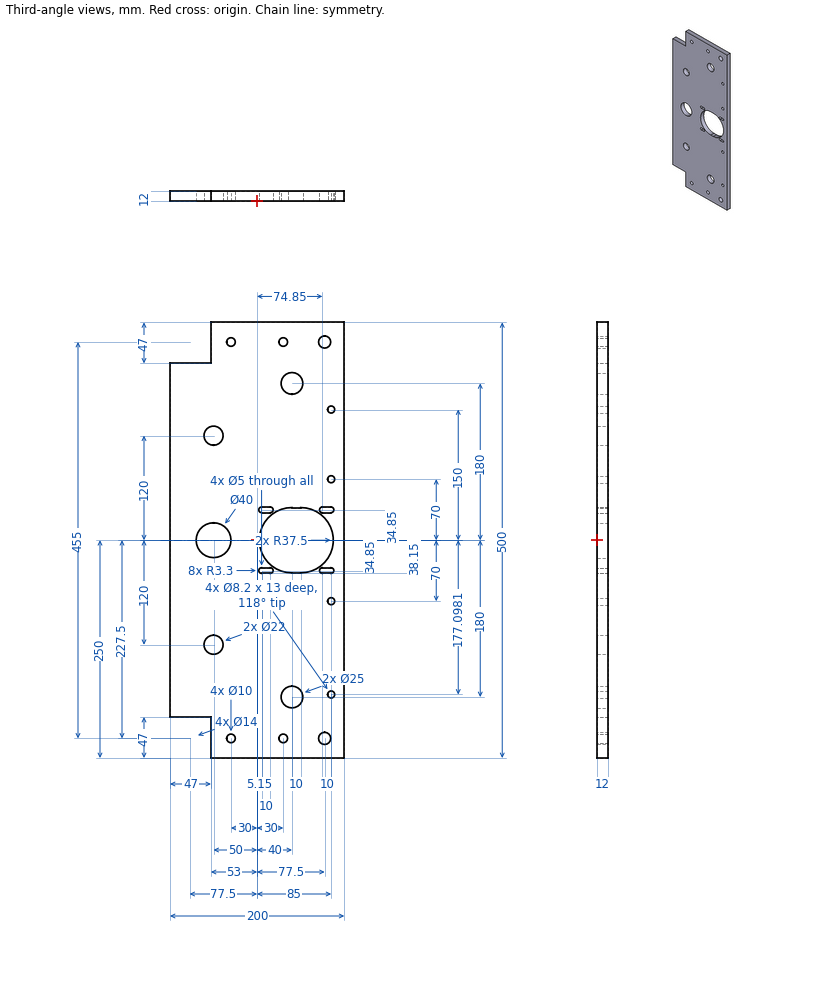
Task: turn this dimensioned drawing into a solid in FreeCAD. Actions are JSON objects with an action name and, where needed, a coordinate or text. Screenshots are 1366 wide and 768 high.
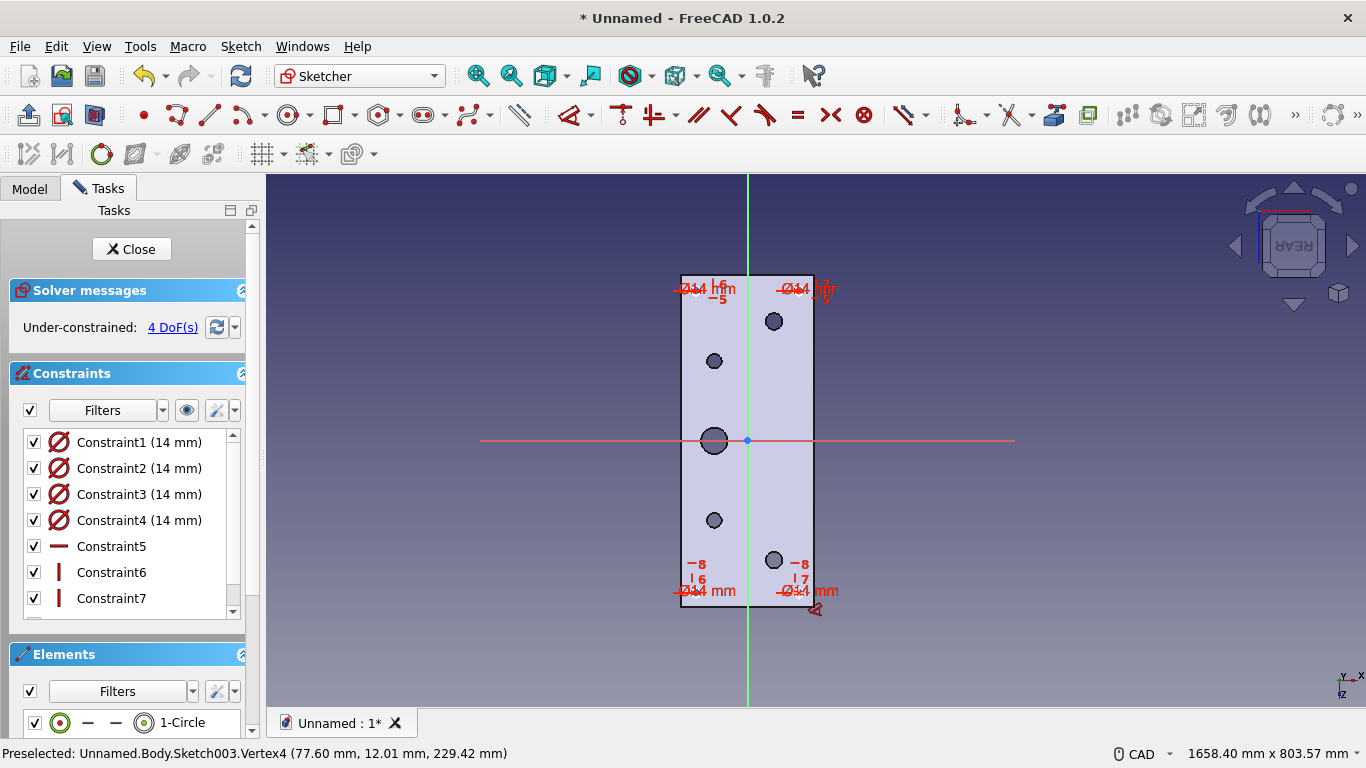
{"action": "left_click", "coordinate": [696, 291]}
{"action": "left_click", "coordinate": [722, 257]}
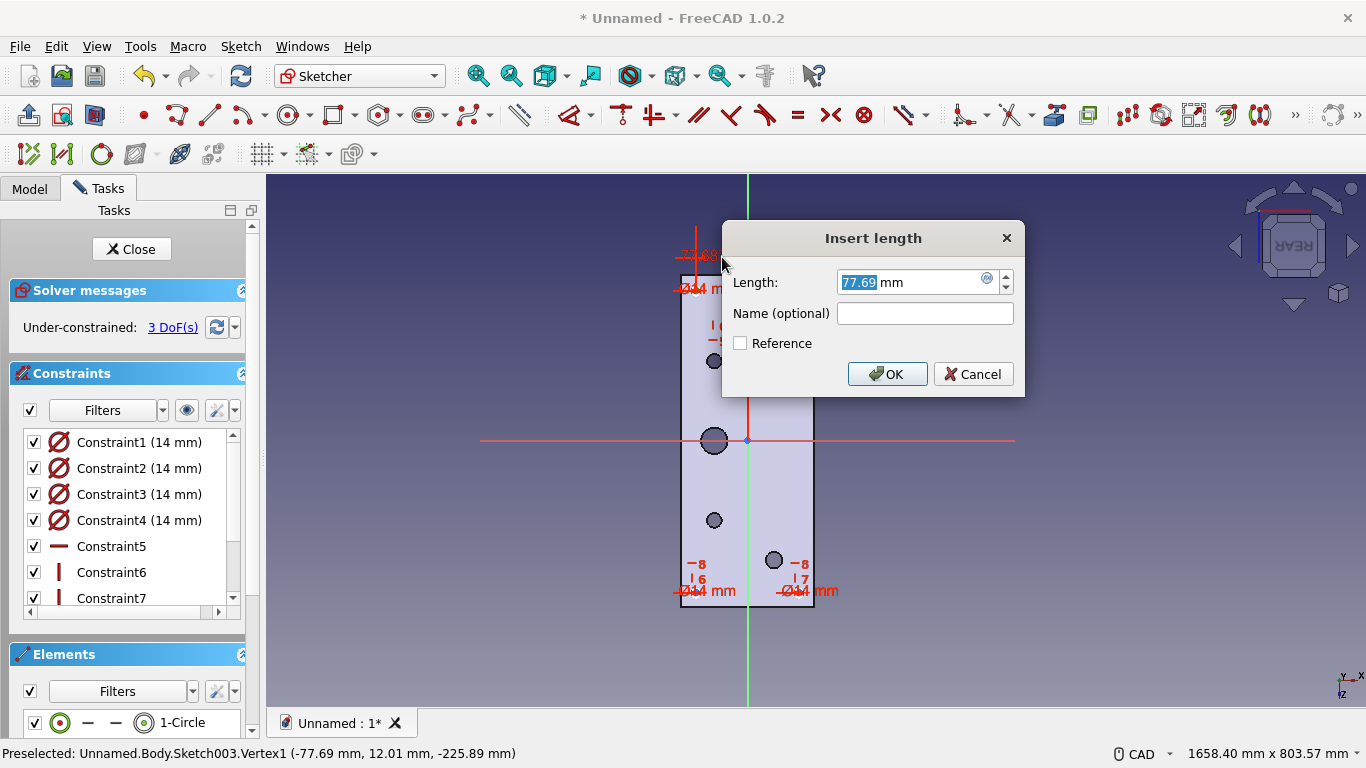
{"action": "type", "text": "77.5"}
{"action": "key", "text": "Return"}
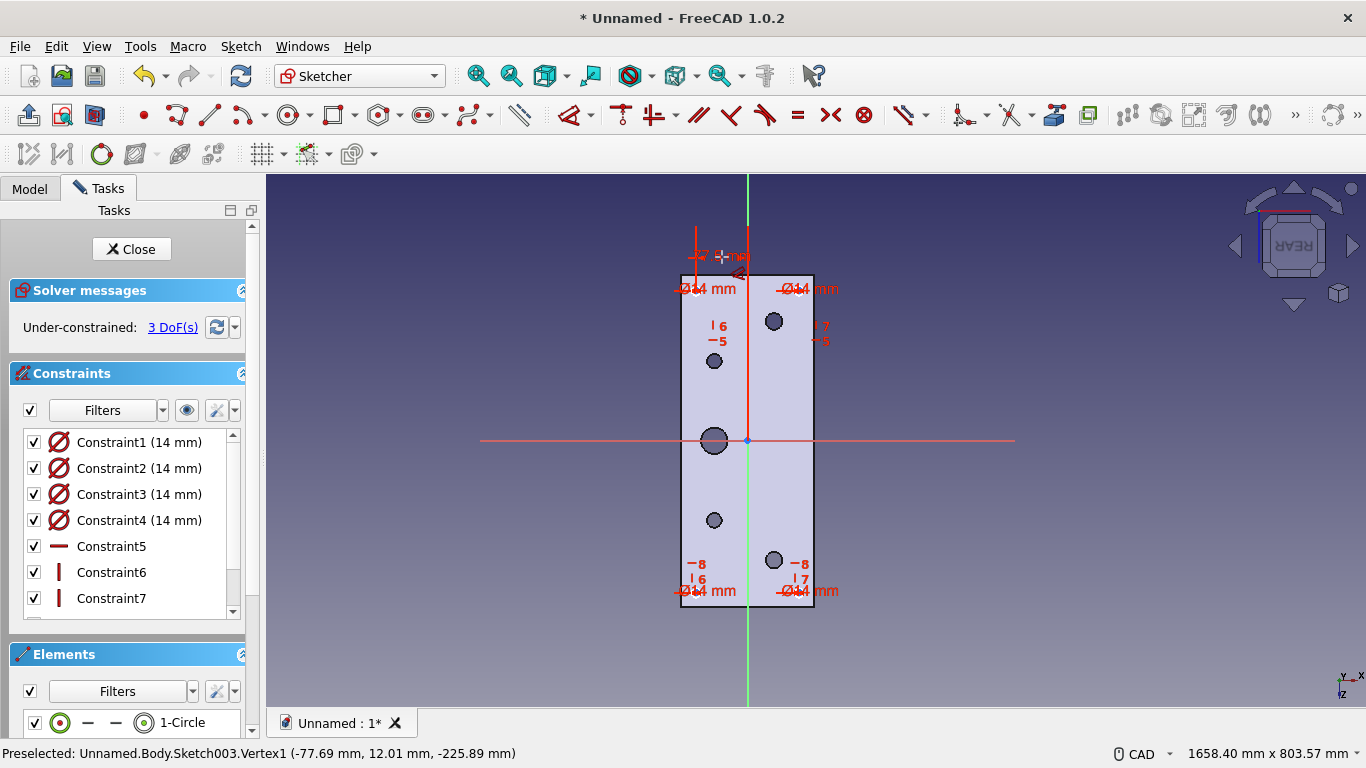
{"action": "left_click", "coordinate": [799, 291]}
{"action": "left_click", "coordinate": [773, 475]}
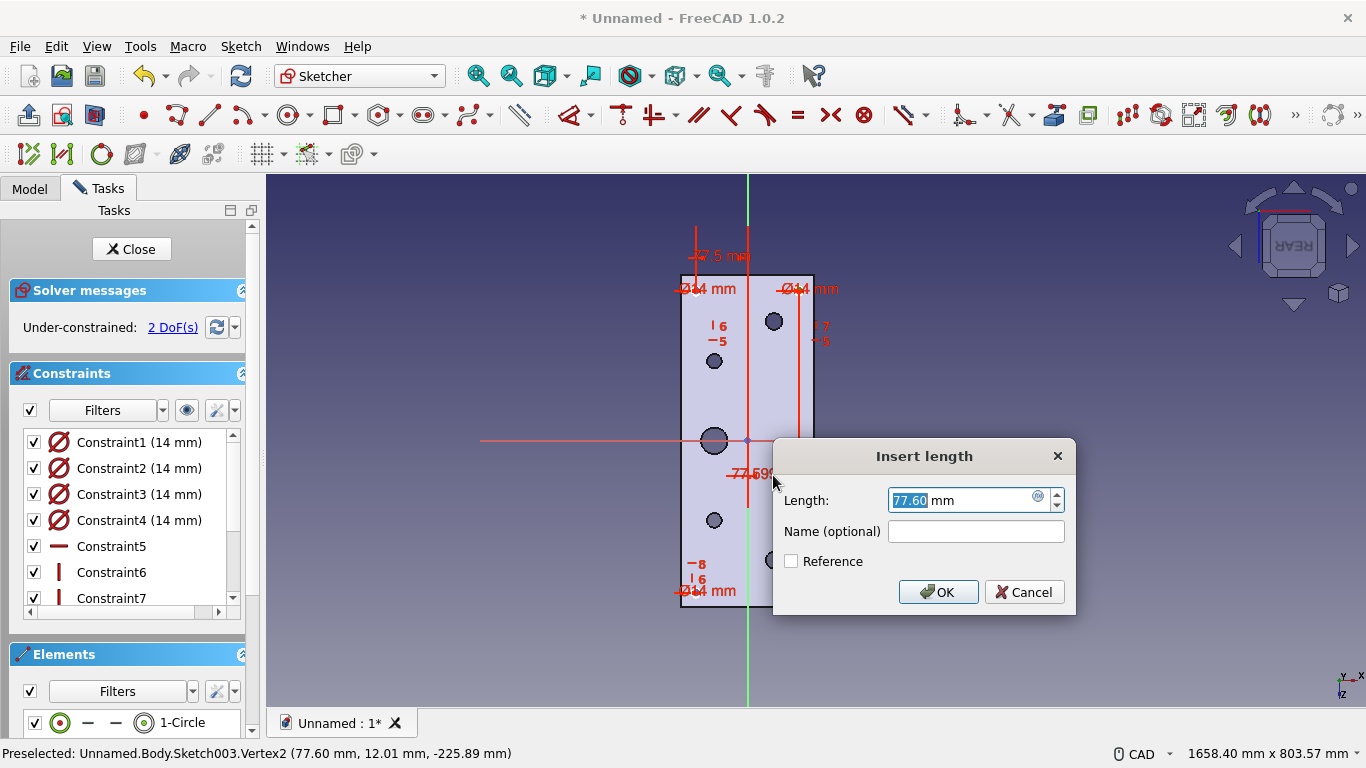
{"action": "type", "text": "77.5"}
{"action": "key", "text": "Return"}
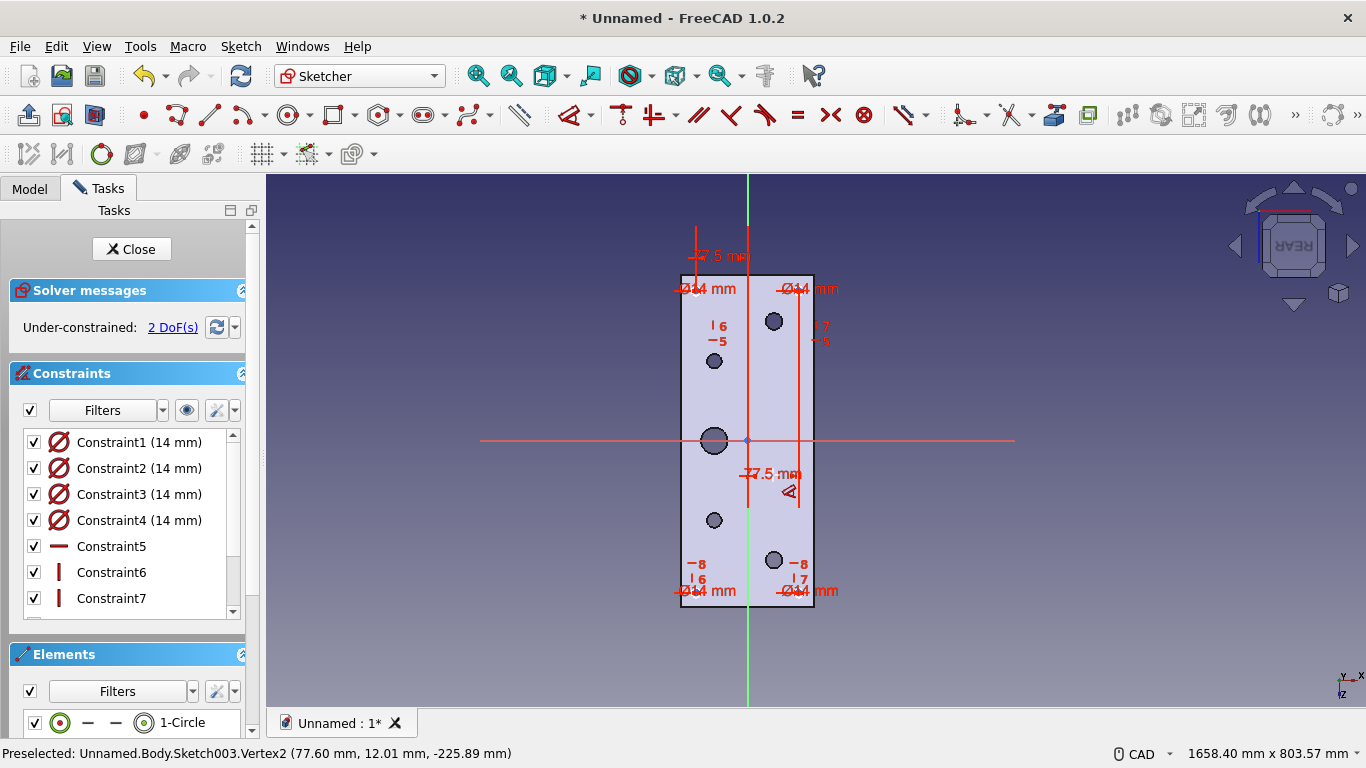
{"action": "left_click", "coordinate": [696, 291]}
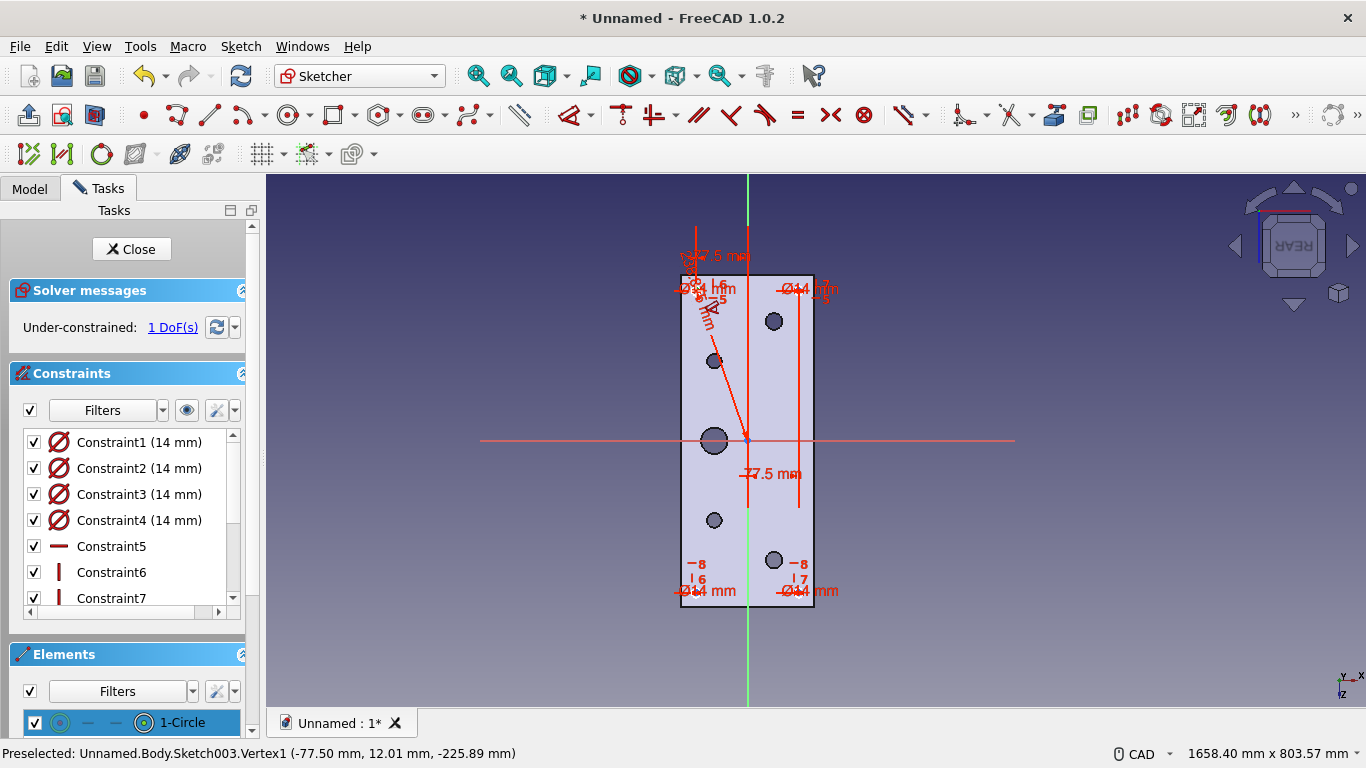
{"action": "left_click", "coordinate": [696, 593]}
{"action": "left_click", "coordinate": [662, 373]}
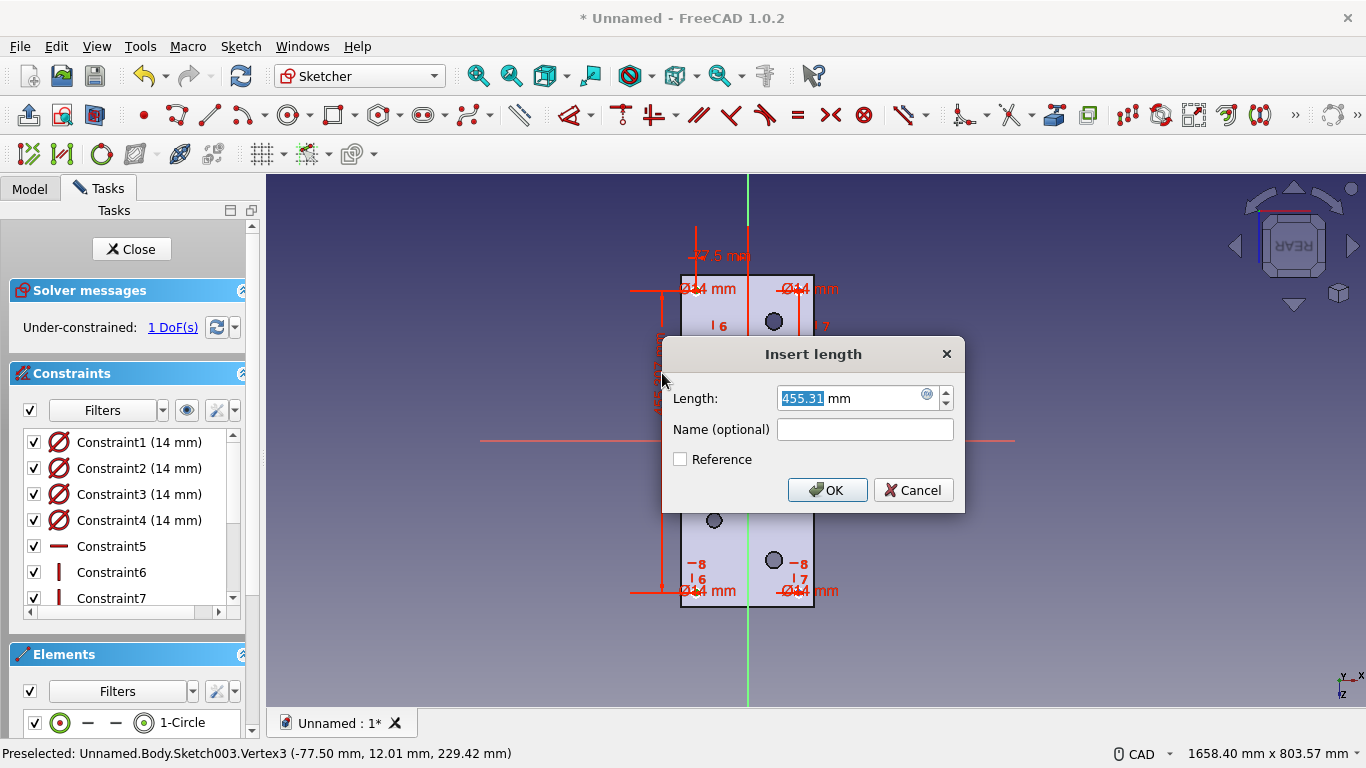
{"action": "type", "text": "455"}
{"action": "key", "text": "Return"}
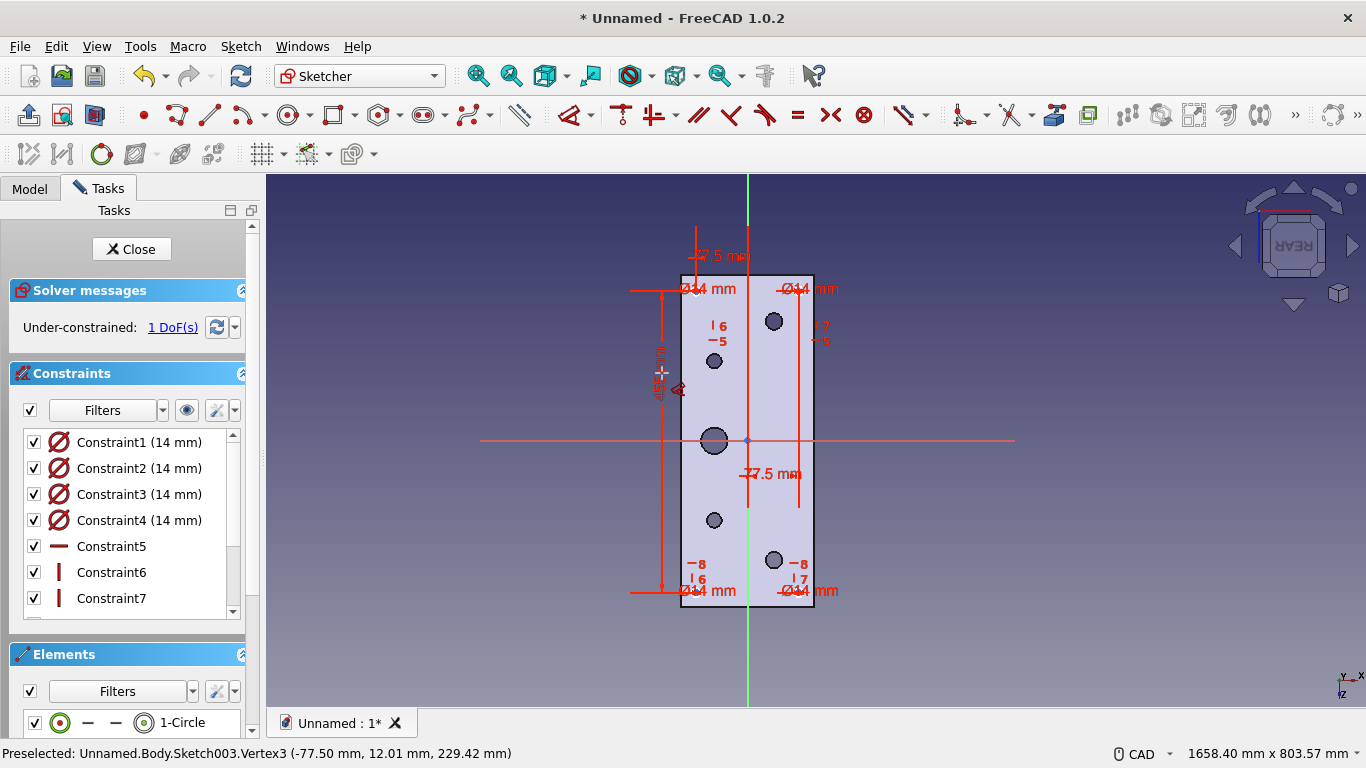
{"action": "left_click", "coordinate": [696, 291]}
{"action": "left_click", "coordinate": [662, 331]}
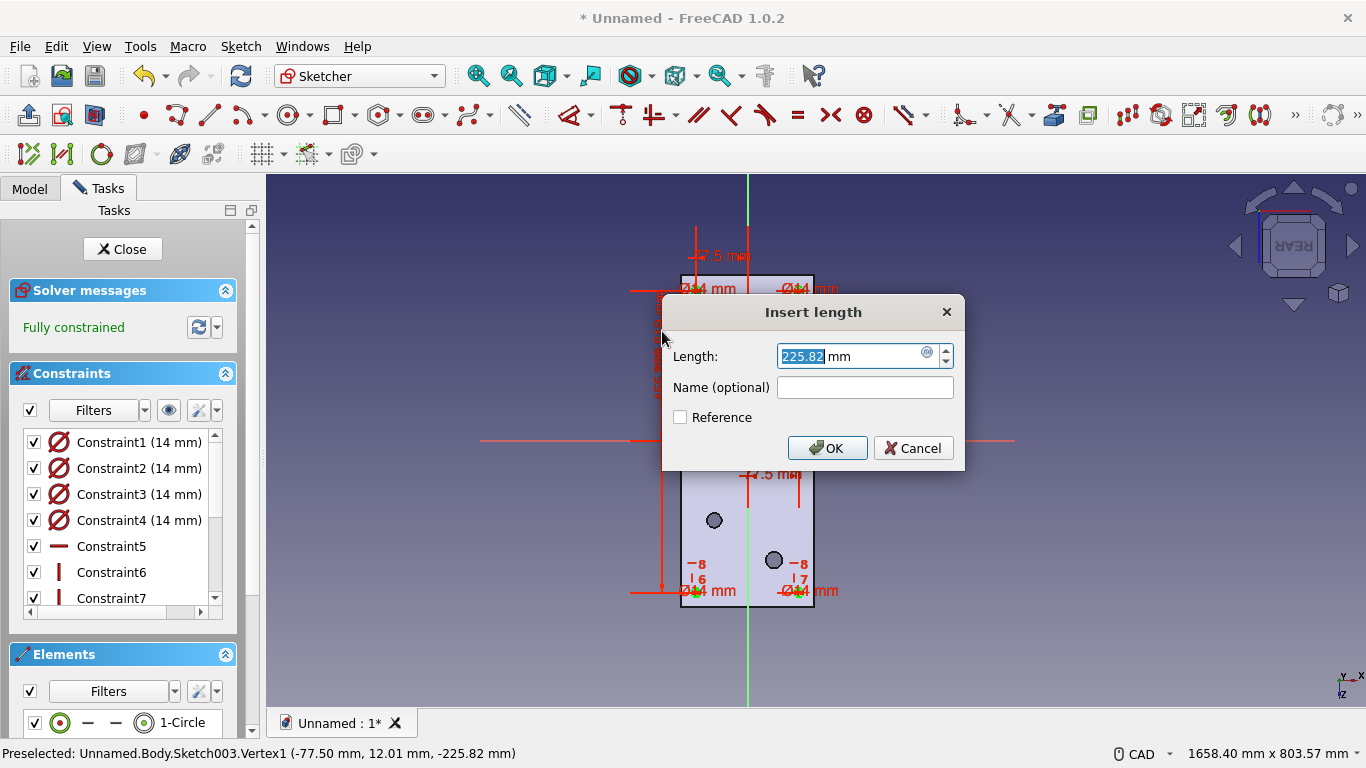
{"action": "type", "text": "227.5"}
{"action": "key", "text": "Return"}
{"action": "key", "text": "Escape"}